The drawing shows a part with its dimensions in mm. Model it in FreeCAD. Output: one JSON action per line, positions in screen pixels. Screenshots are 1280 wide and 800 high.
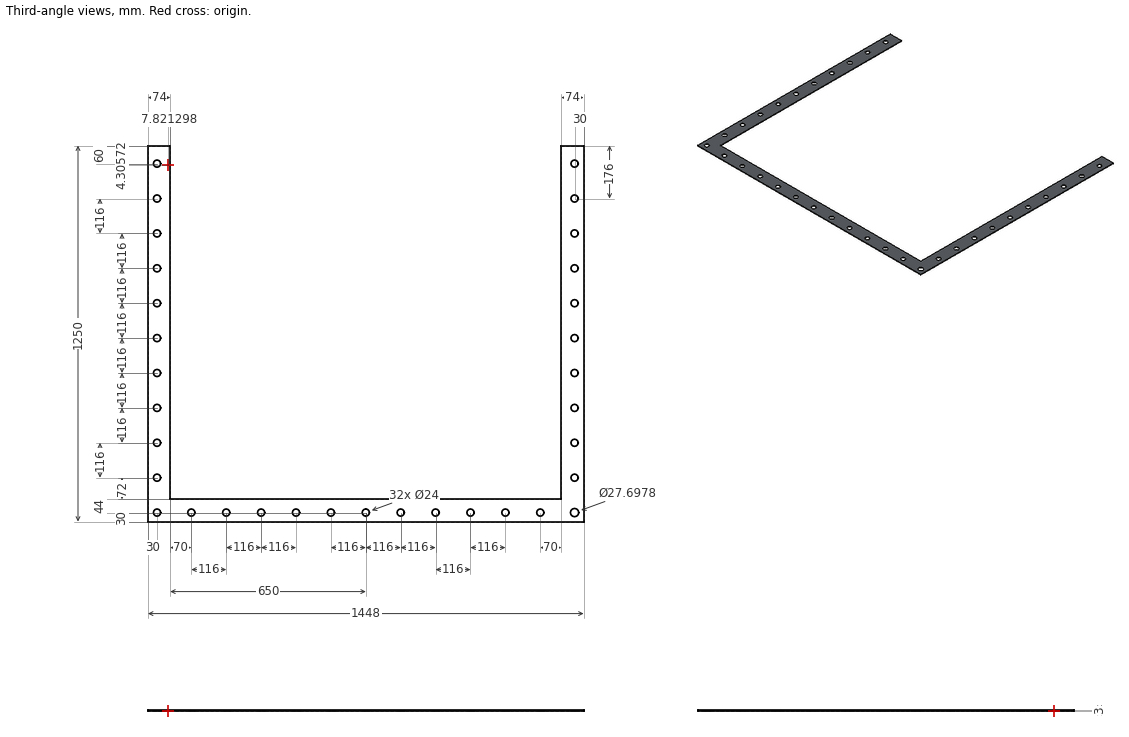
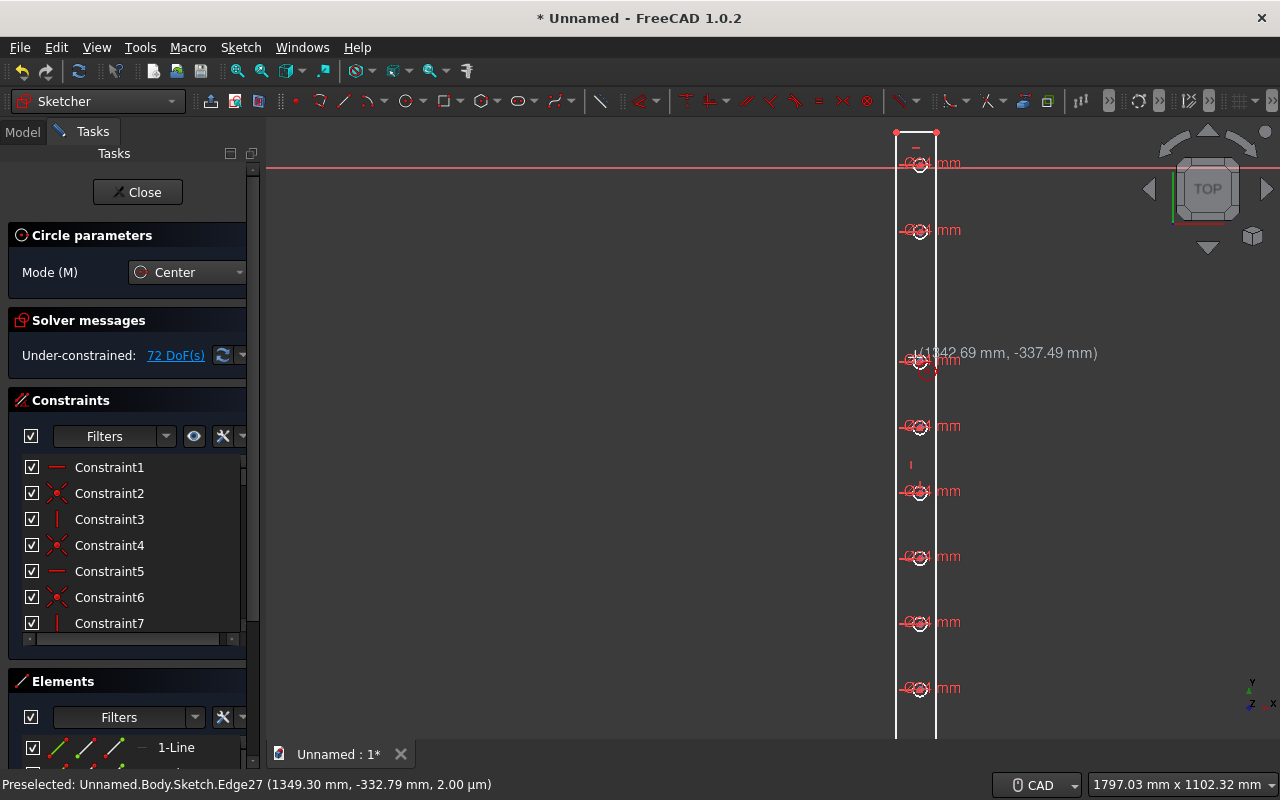
{"action": "scroll", "coordinate": [920, 296], "scroll_direction": "up", "scroll_amount": 7}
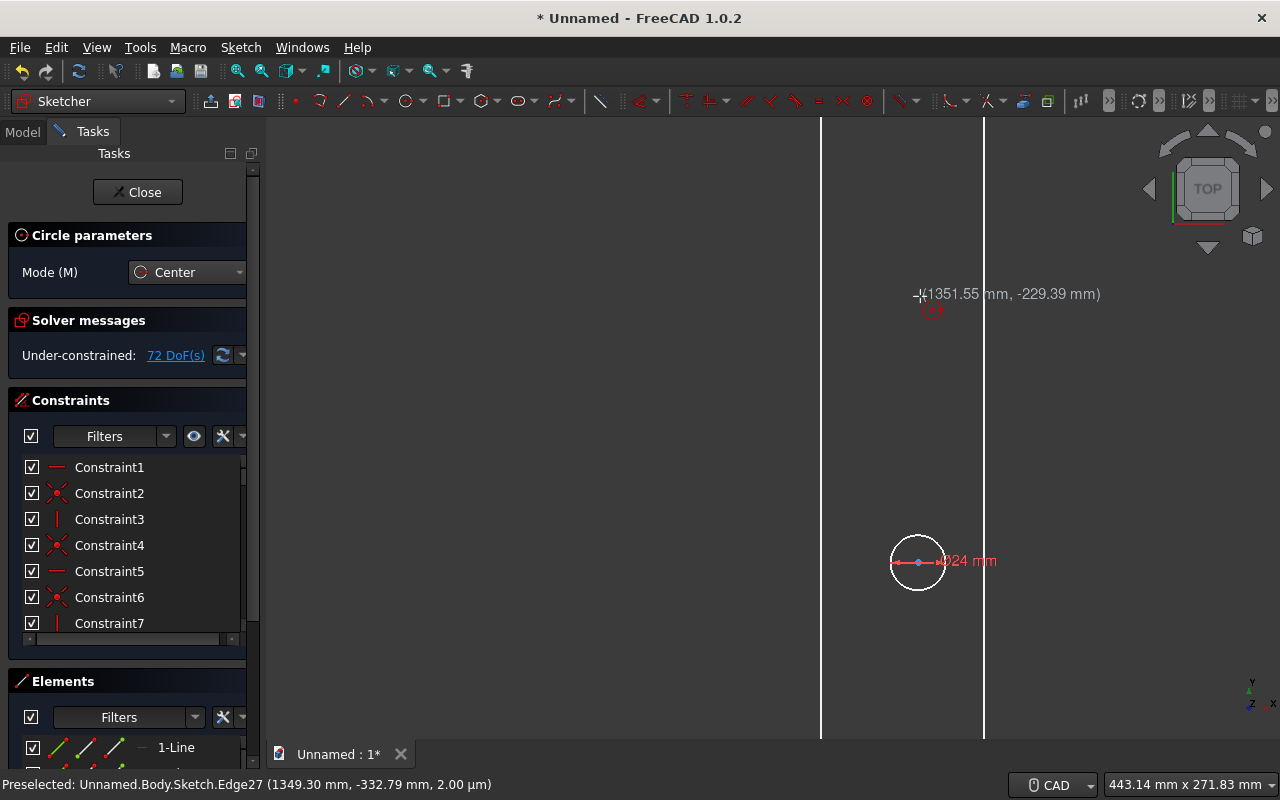
{"action": "scroll", "coordinate": [920, 330], "scroll_direction": "down", "scroll_amount": 10}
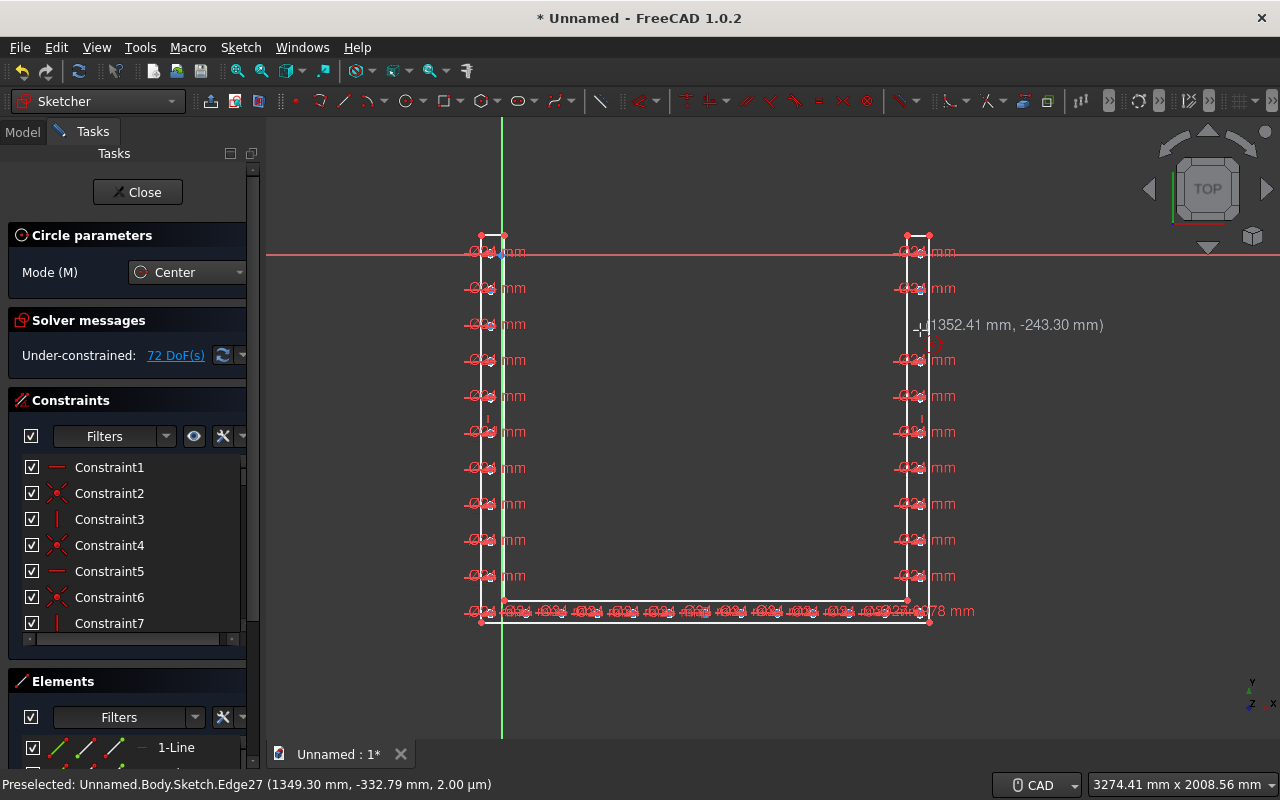
{"action": "scroll", "coordinate": [920, 326], "scroll_direction": "up", "scroll_amount": 3}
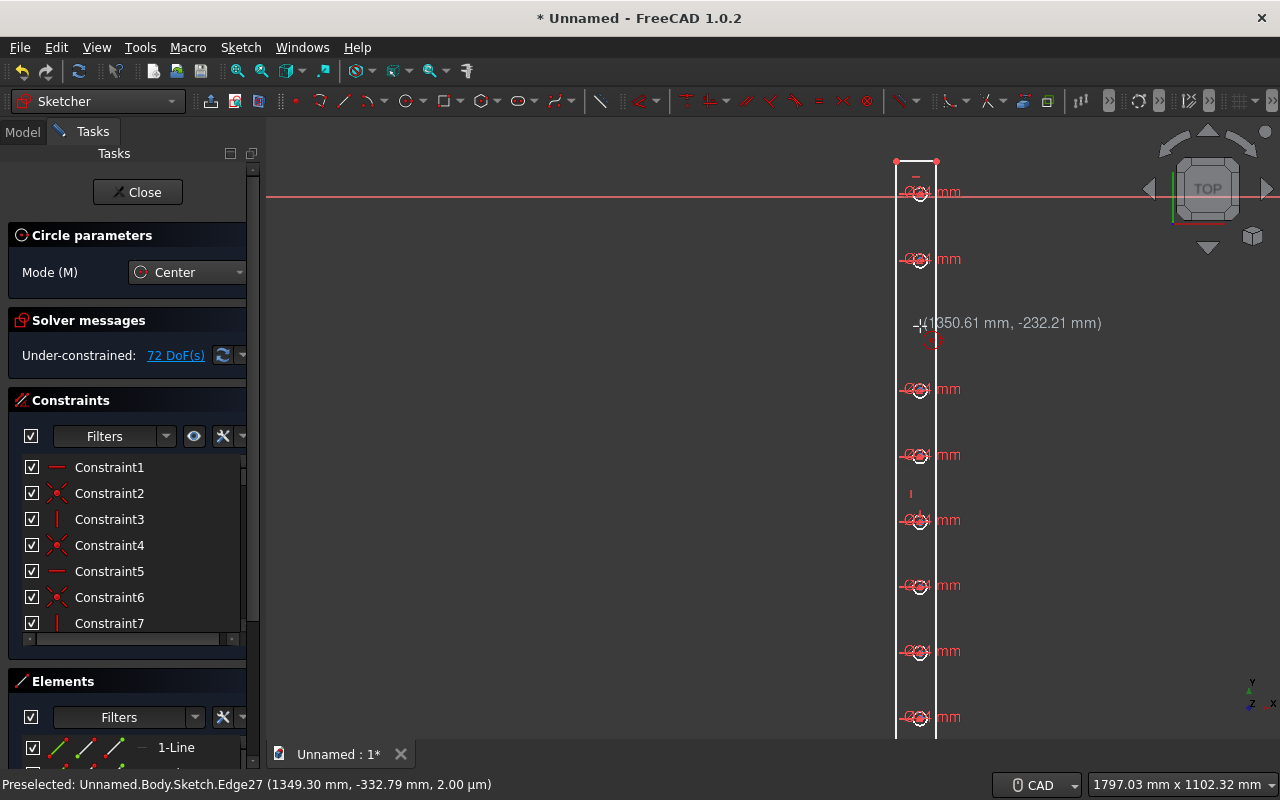
{"action": "left_click", "coordinate": [920, 325]}
{"action": "mouse_move", "coordinate": [915, 320]}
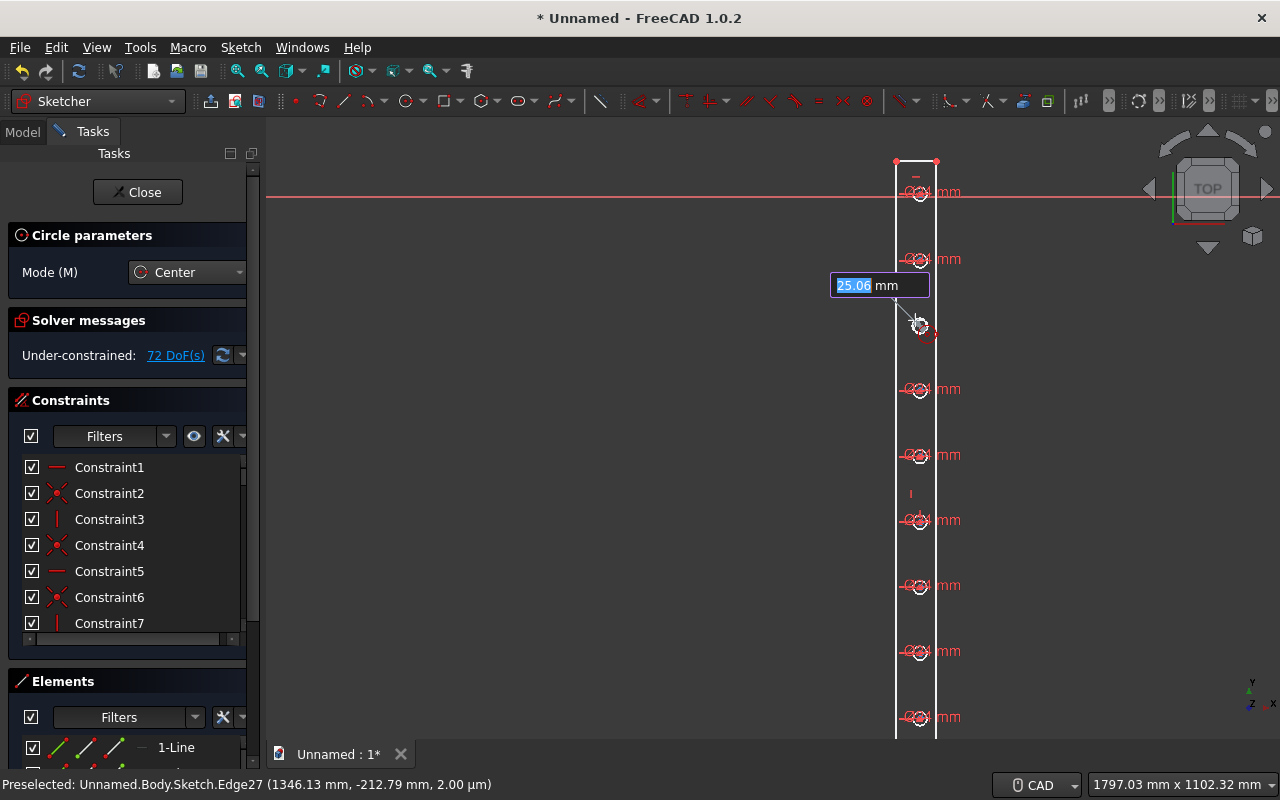
{"action": "type", "text": "24"}
{"action": "key", "text": "Return"}
{"action": "key", "text": "Escape"}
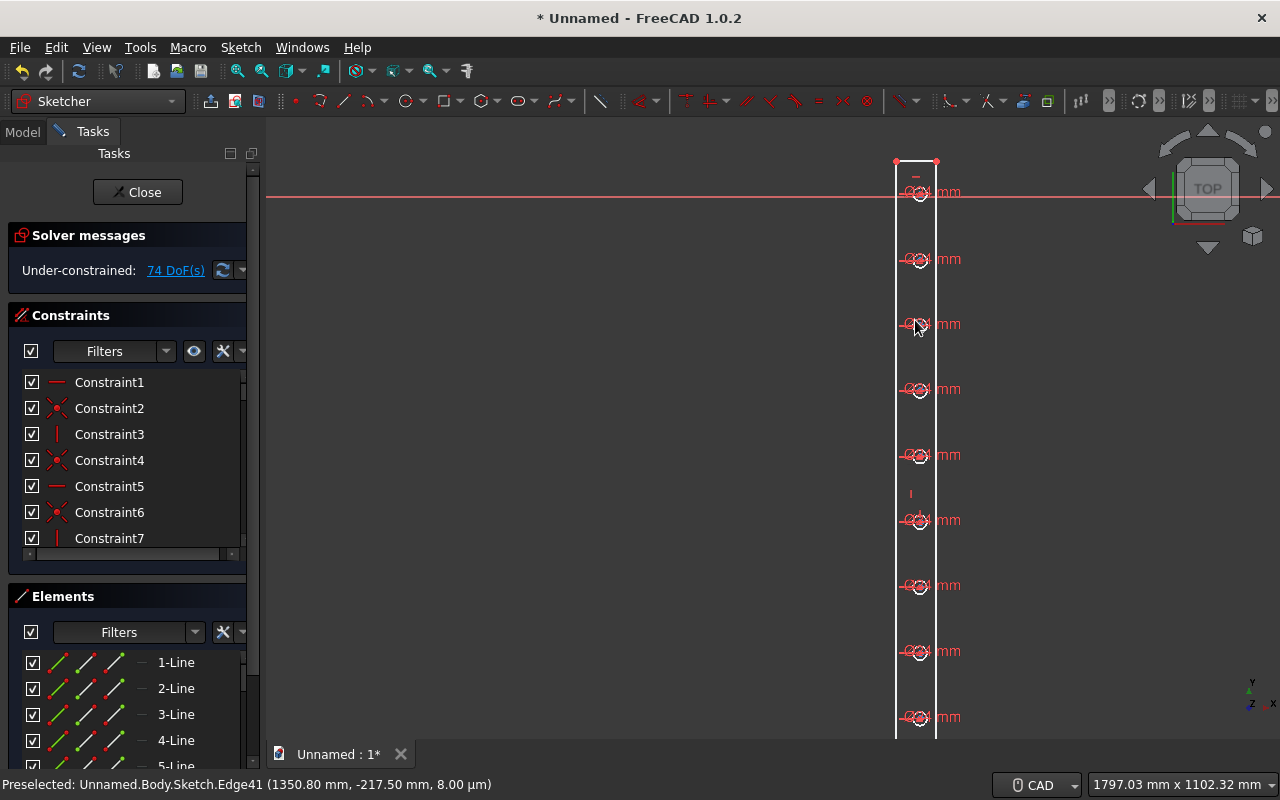
{"action": "scroll", "coordinate": [919, 325], "scroll_direction": "down", "scroll_amount": 3}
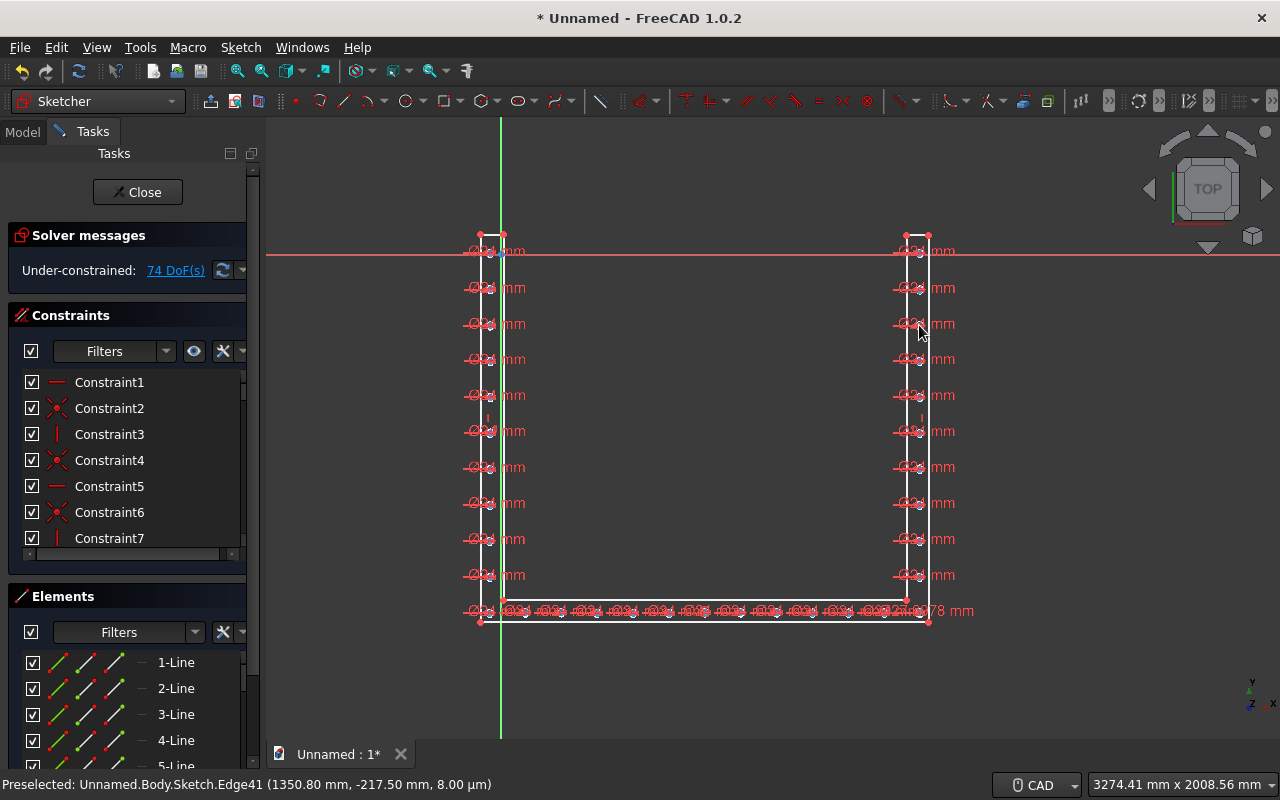
{"action": "left_click", "coordinate": [705, 613]}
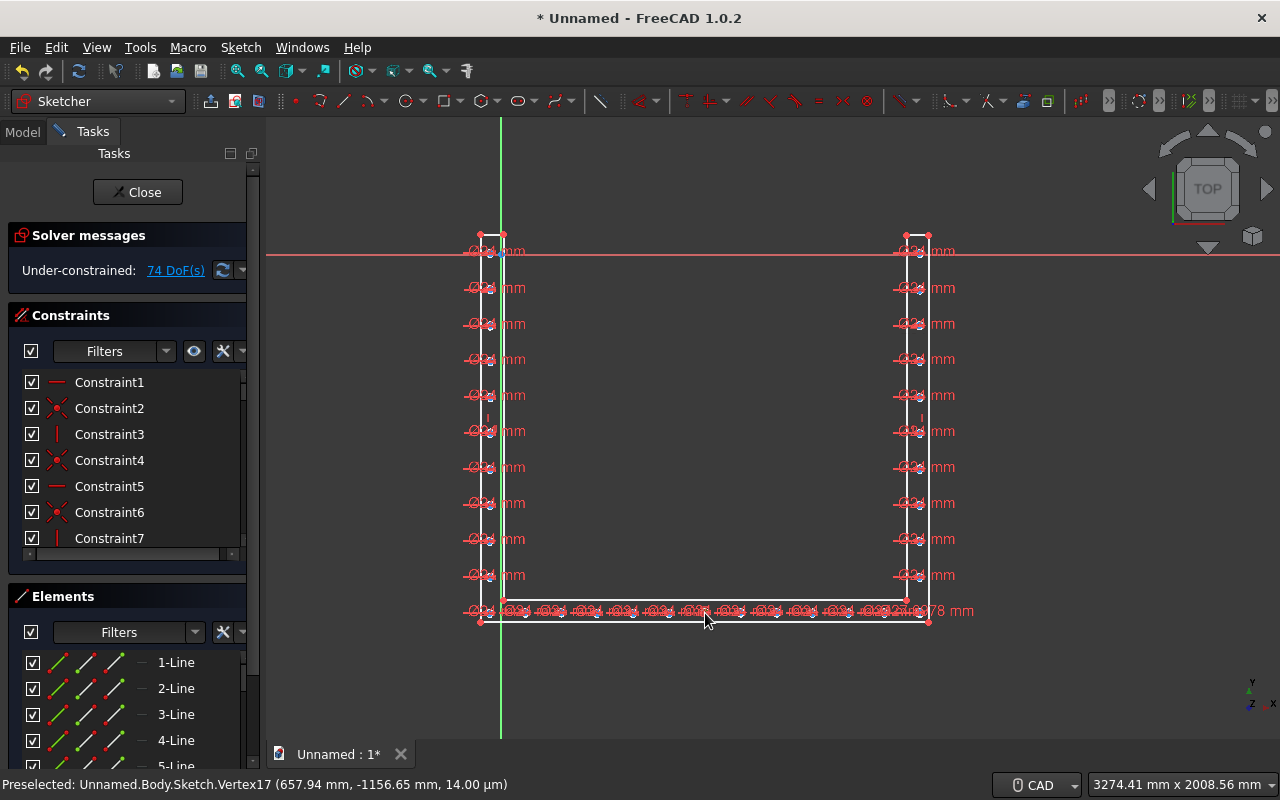
{"action": "left_click", "coordinate": [490, 613]}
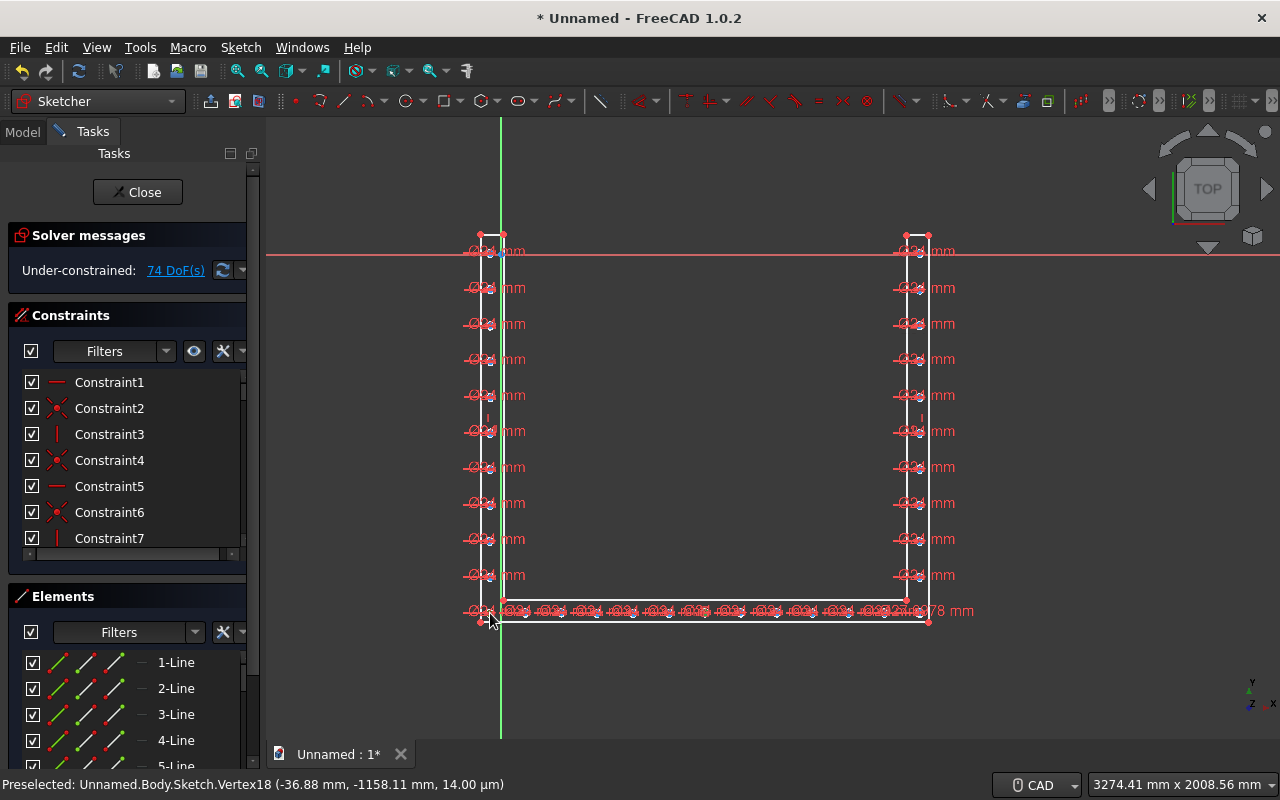
{"action": "key", "text": "h"}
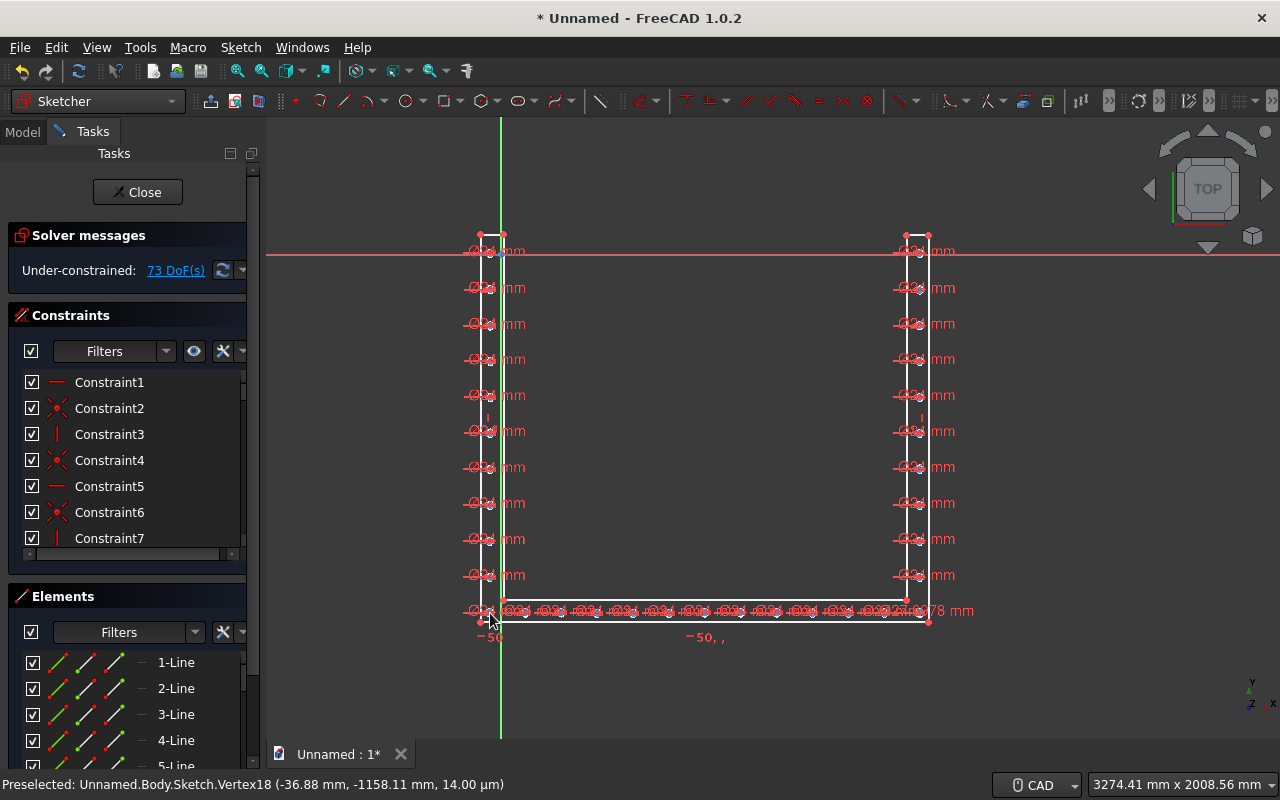
{"action": "left_click", "coordinate": [490, 613]}